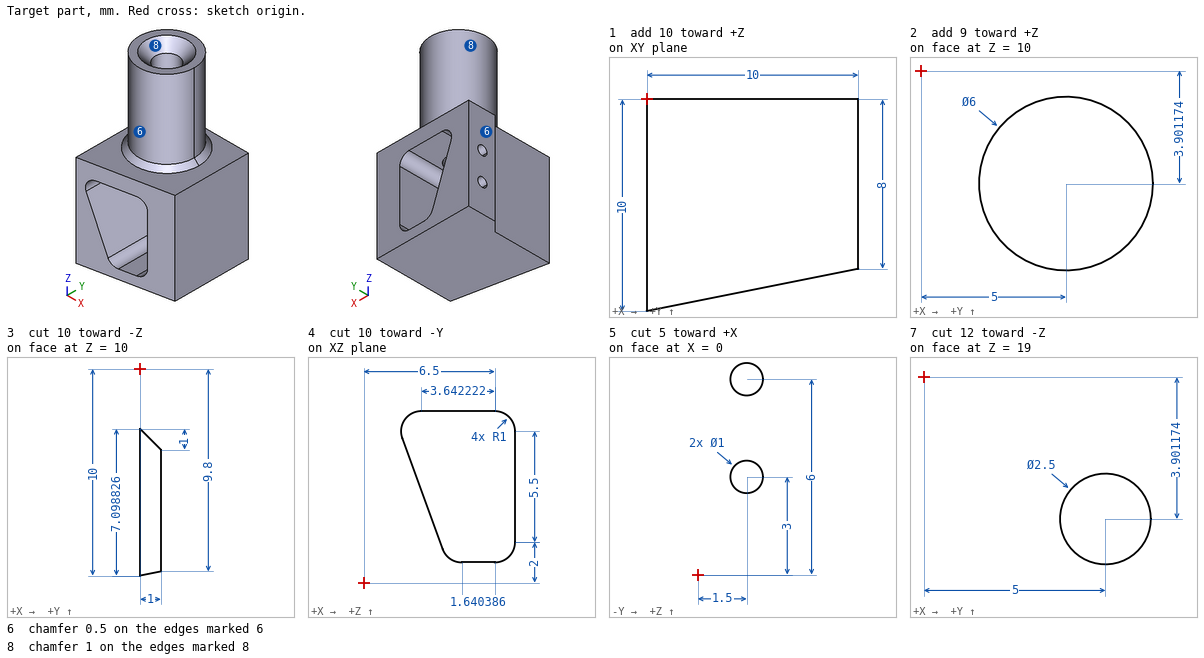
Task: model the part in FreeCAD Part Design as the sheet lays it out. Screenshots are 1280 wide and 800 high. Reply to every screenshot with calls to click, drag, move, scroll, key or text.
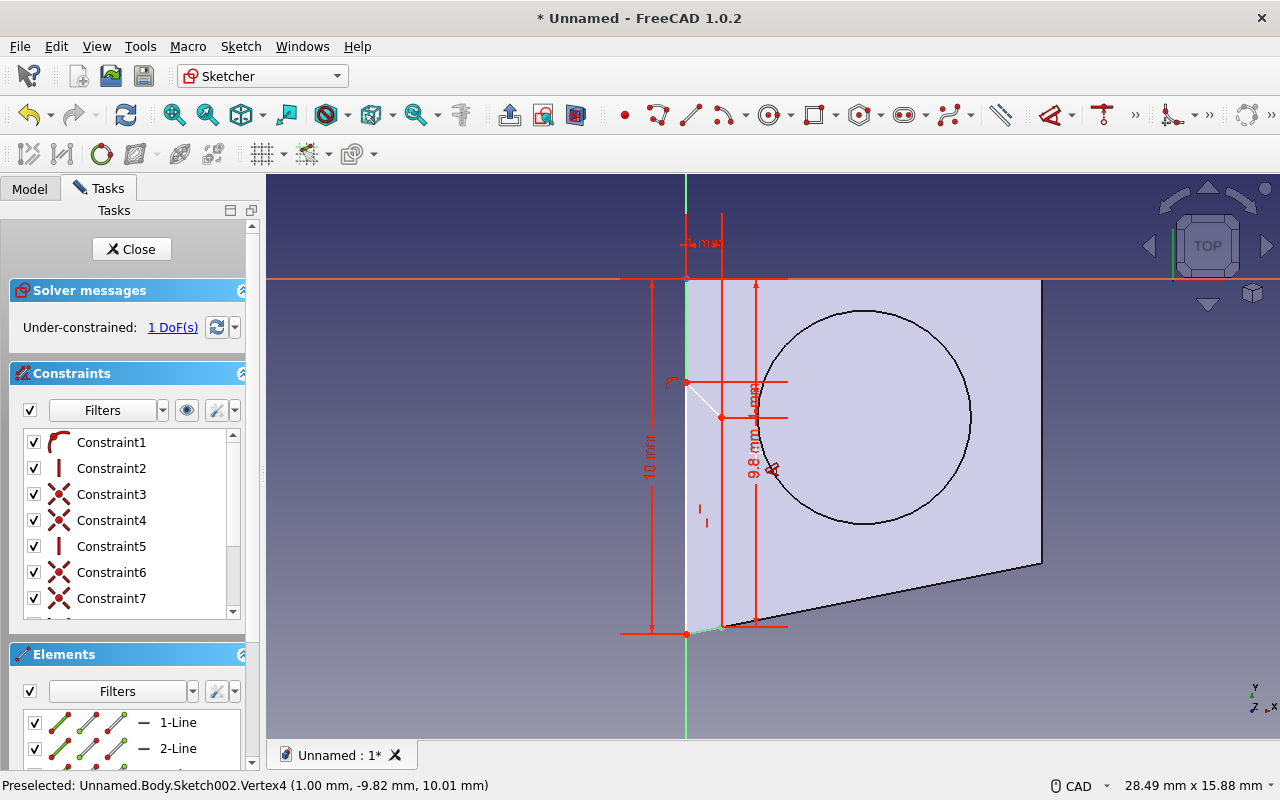
click(686, 458)
click(652, 508)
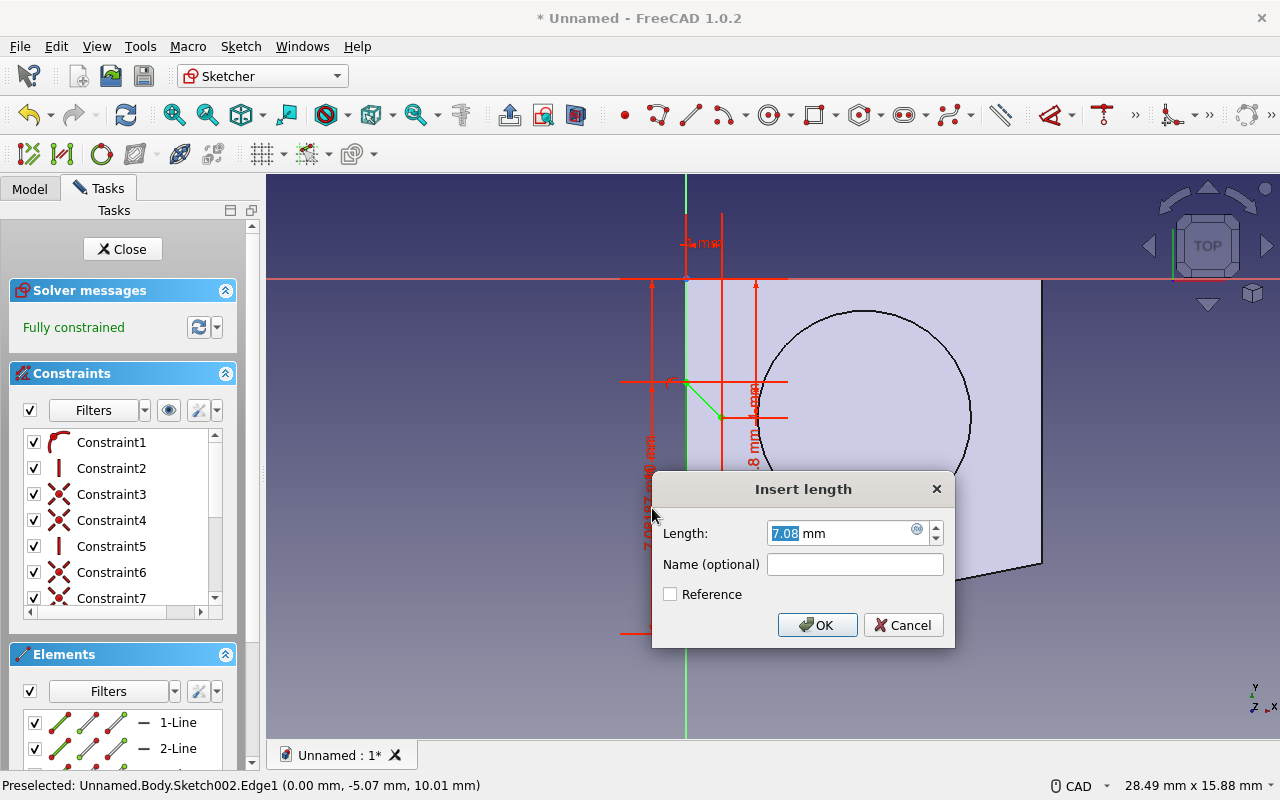
text(7.098826)
key(Return)
key(Escape)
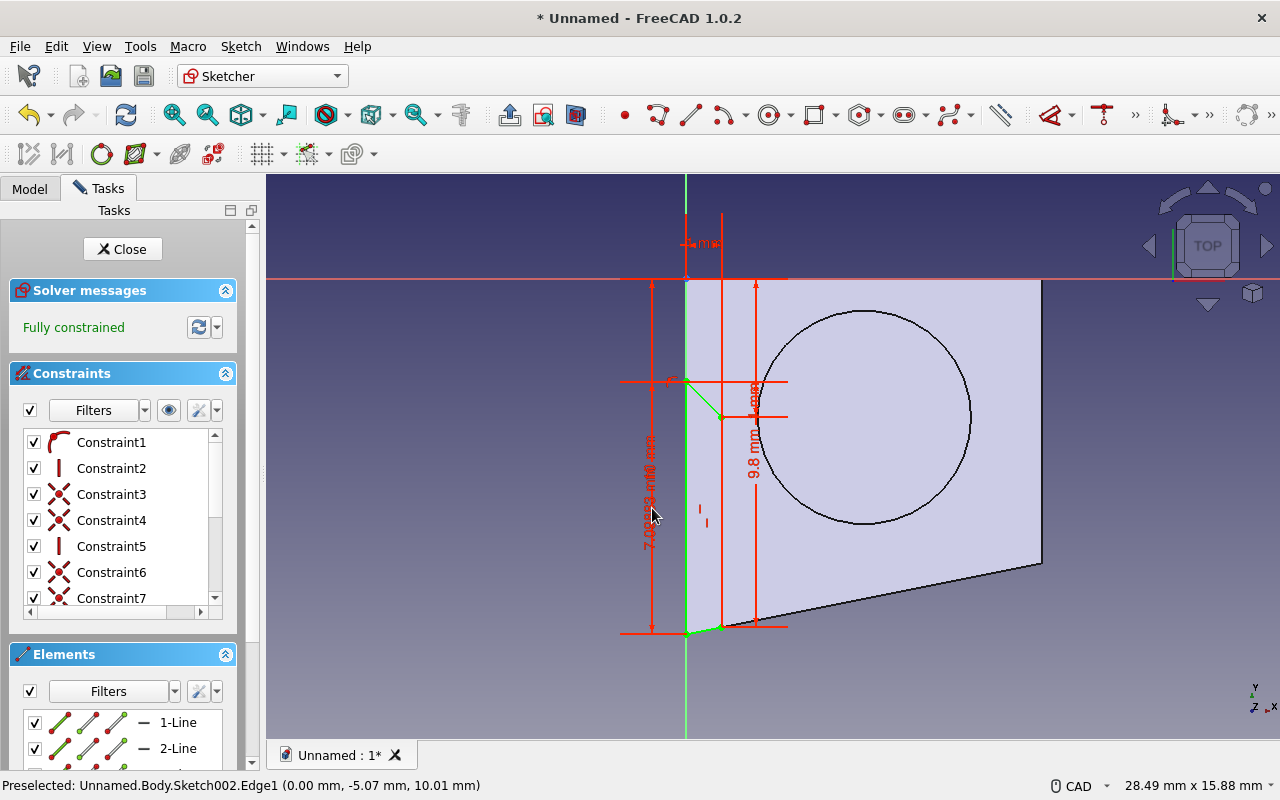
click(123, 249)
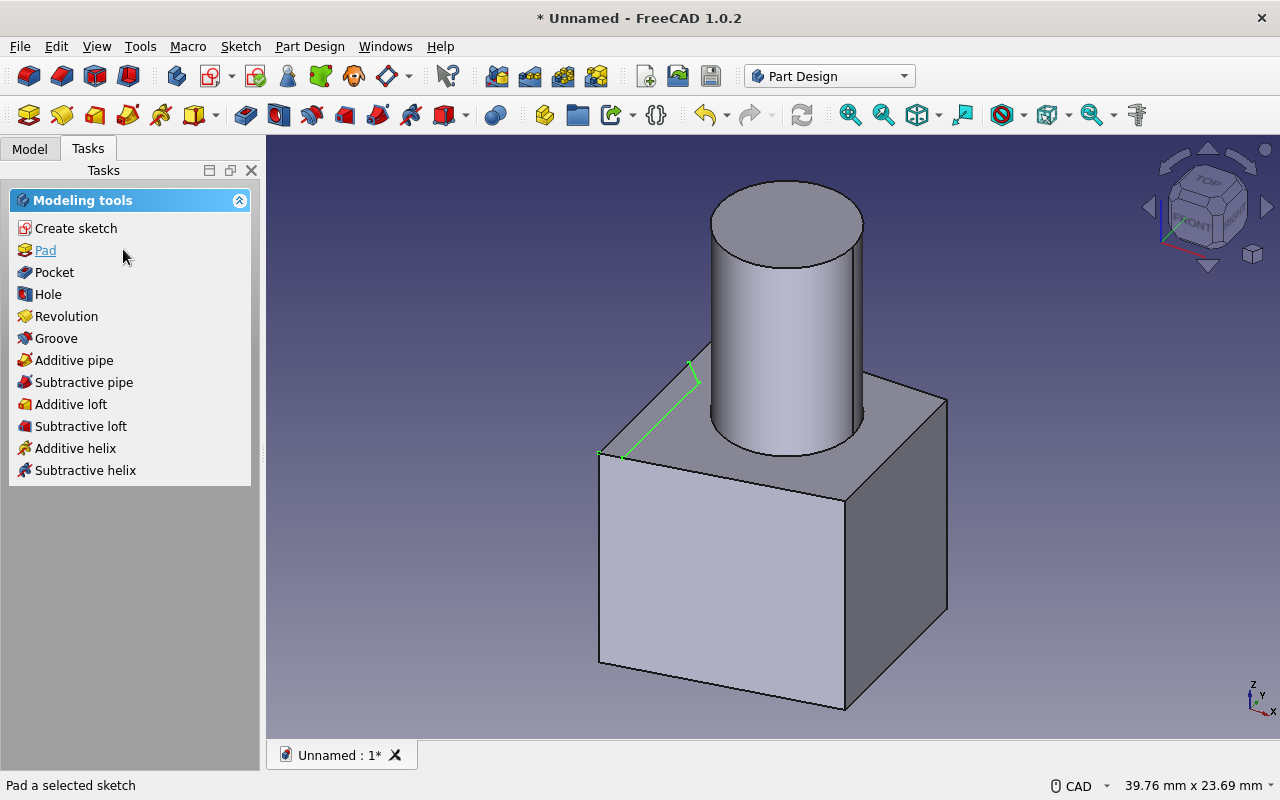
click(246, 116)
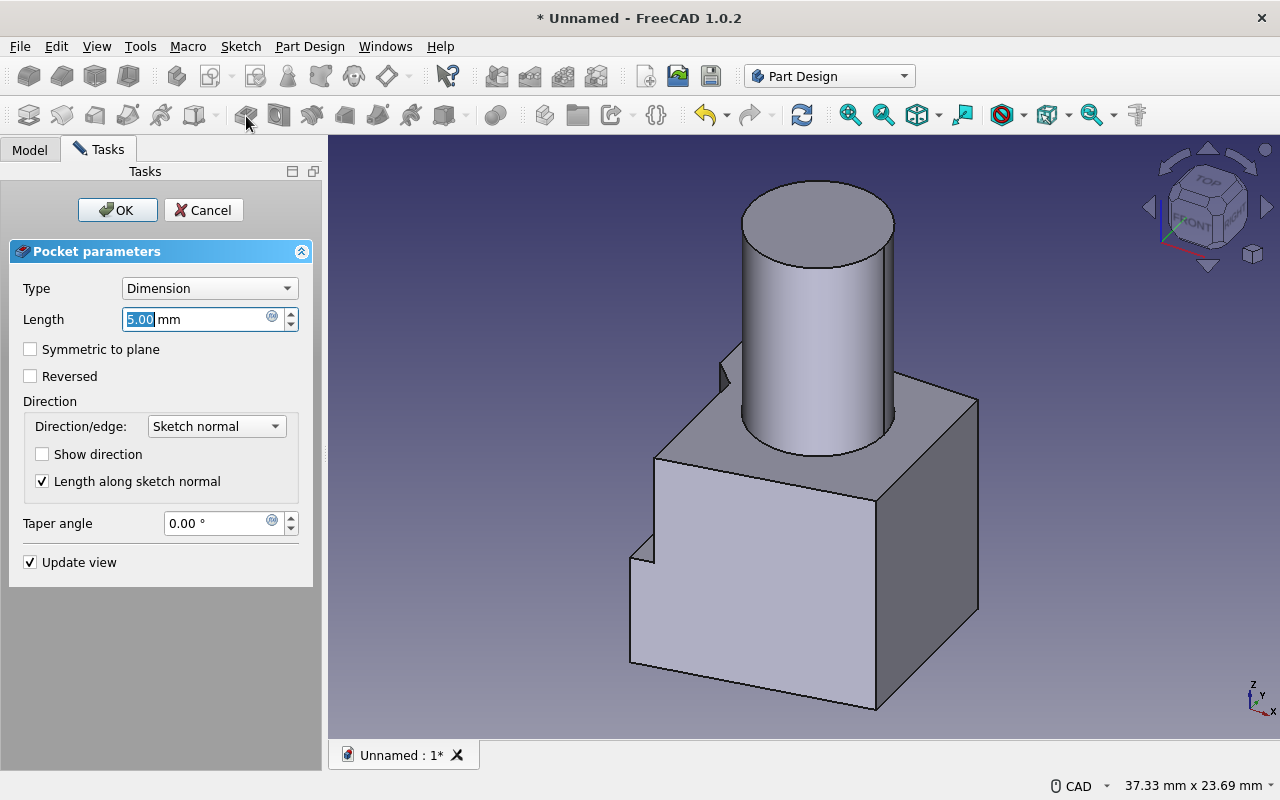
text(10)
key(Tab)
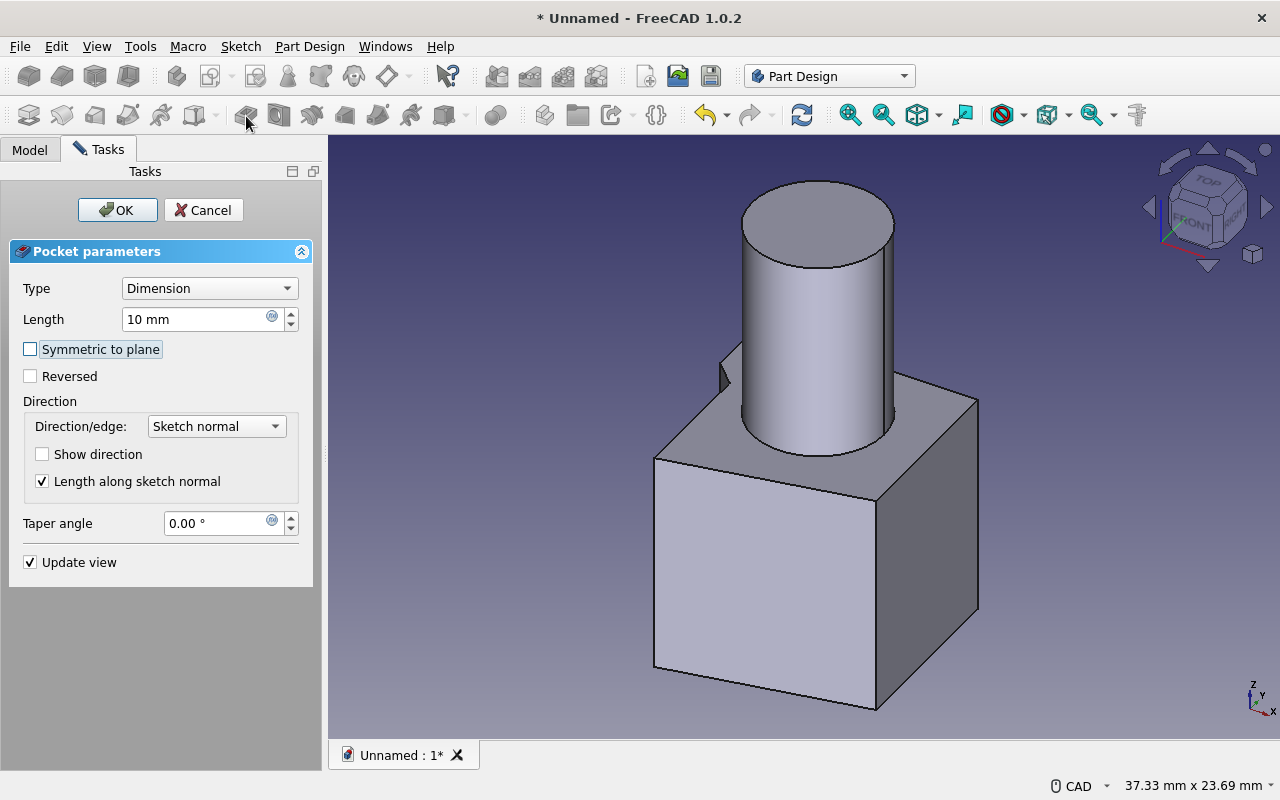
click(118, 210)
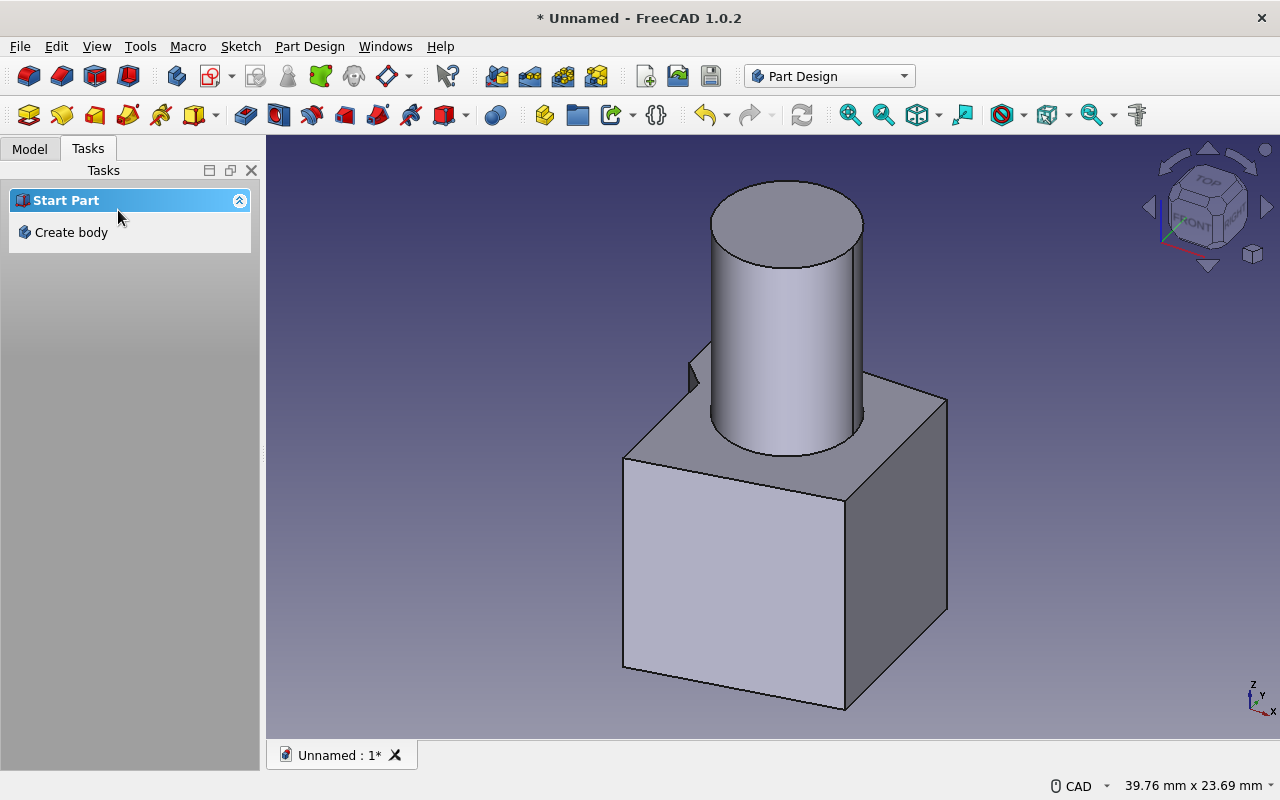
click(210, 76)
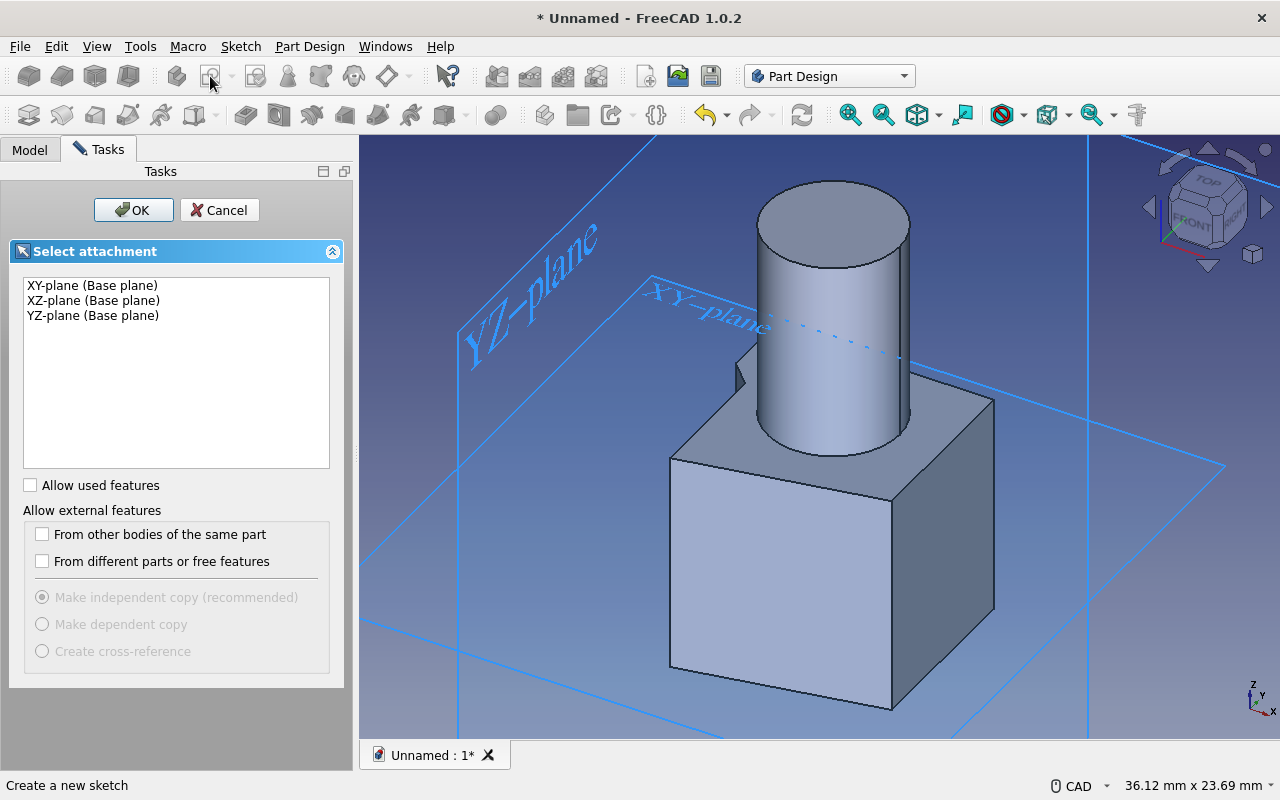
click(84, 300)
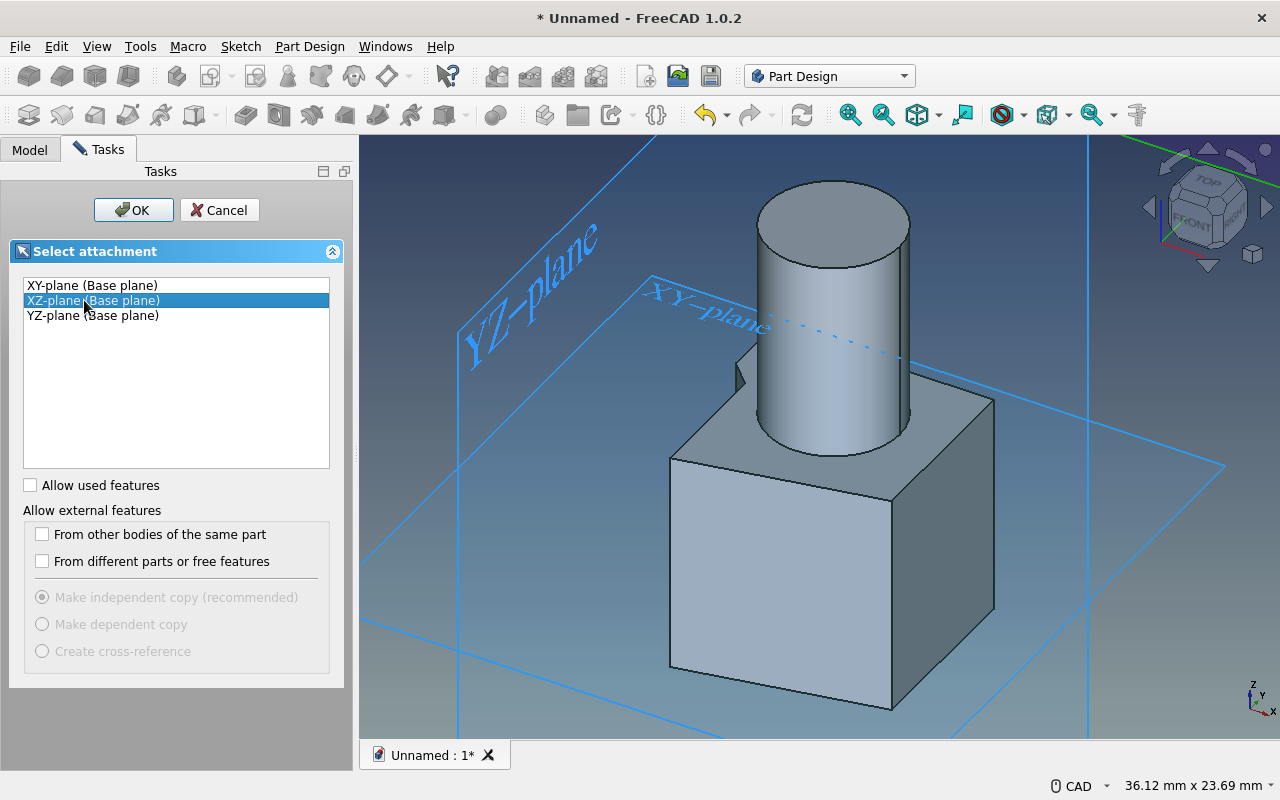
click(134, 210)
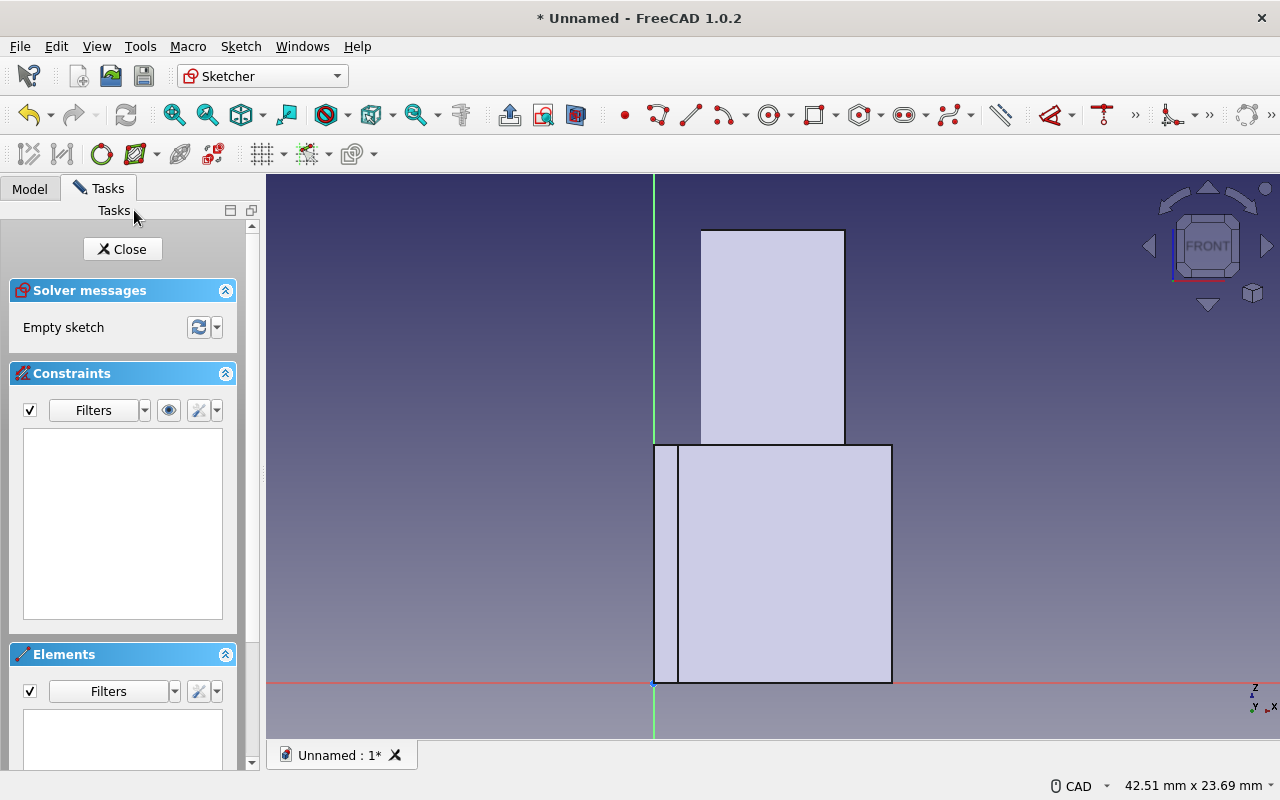
click(576, 116)